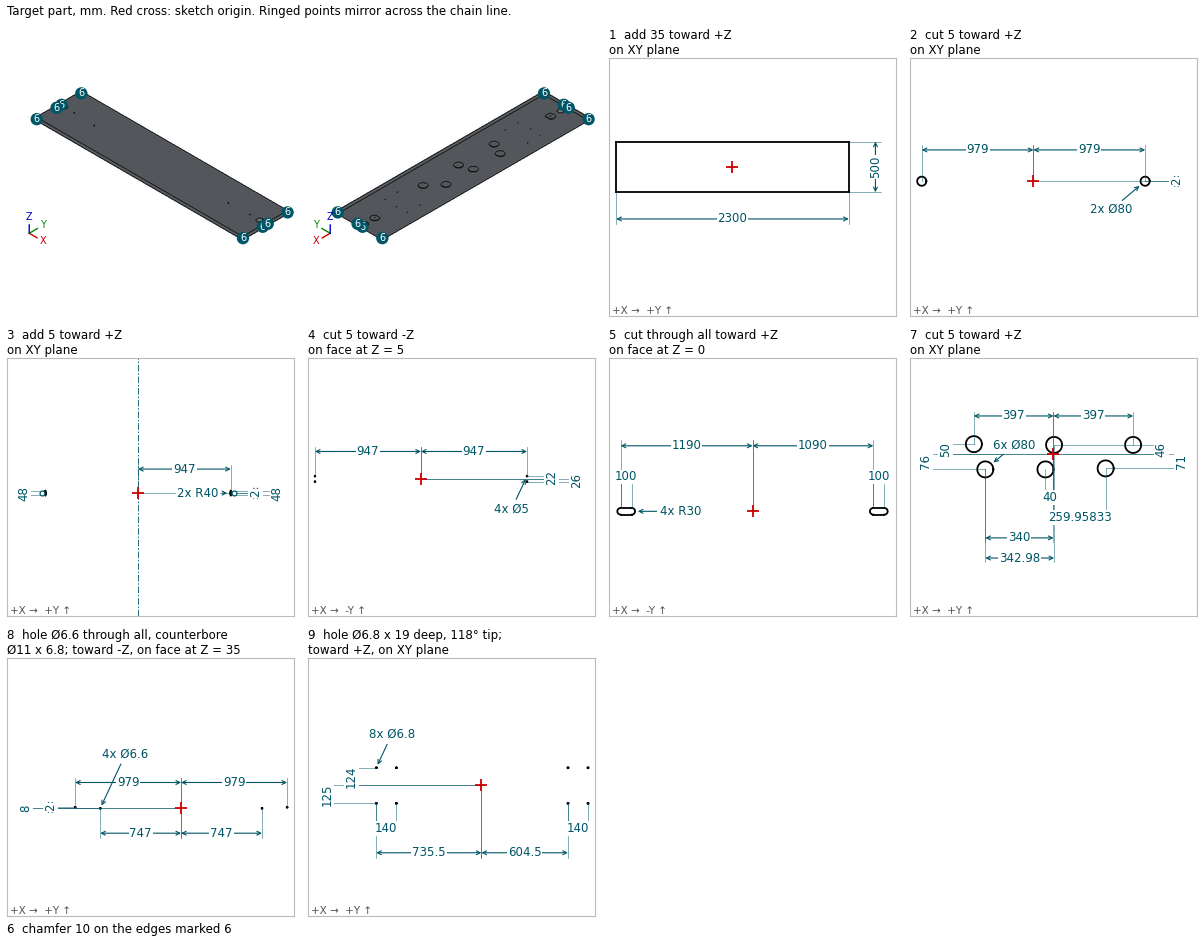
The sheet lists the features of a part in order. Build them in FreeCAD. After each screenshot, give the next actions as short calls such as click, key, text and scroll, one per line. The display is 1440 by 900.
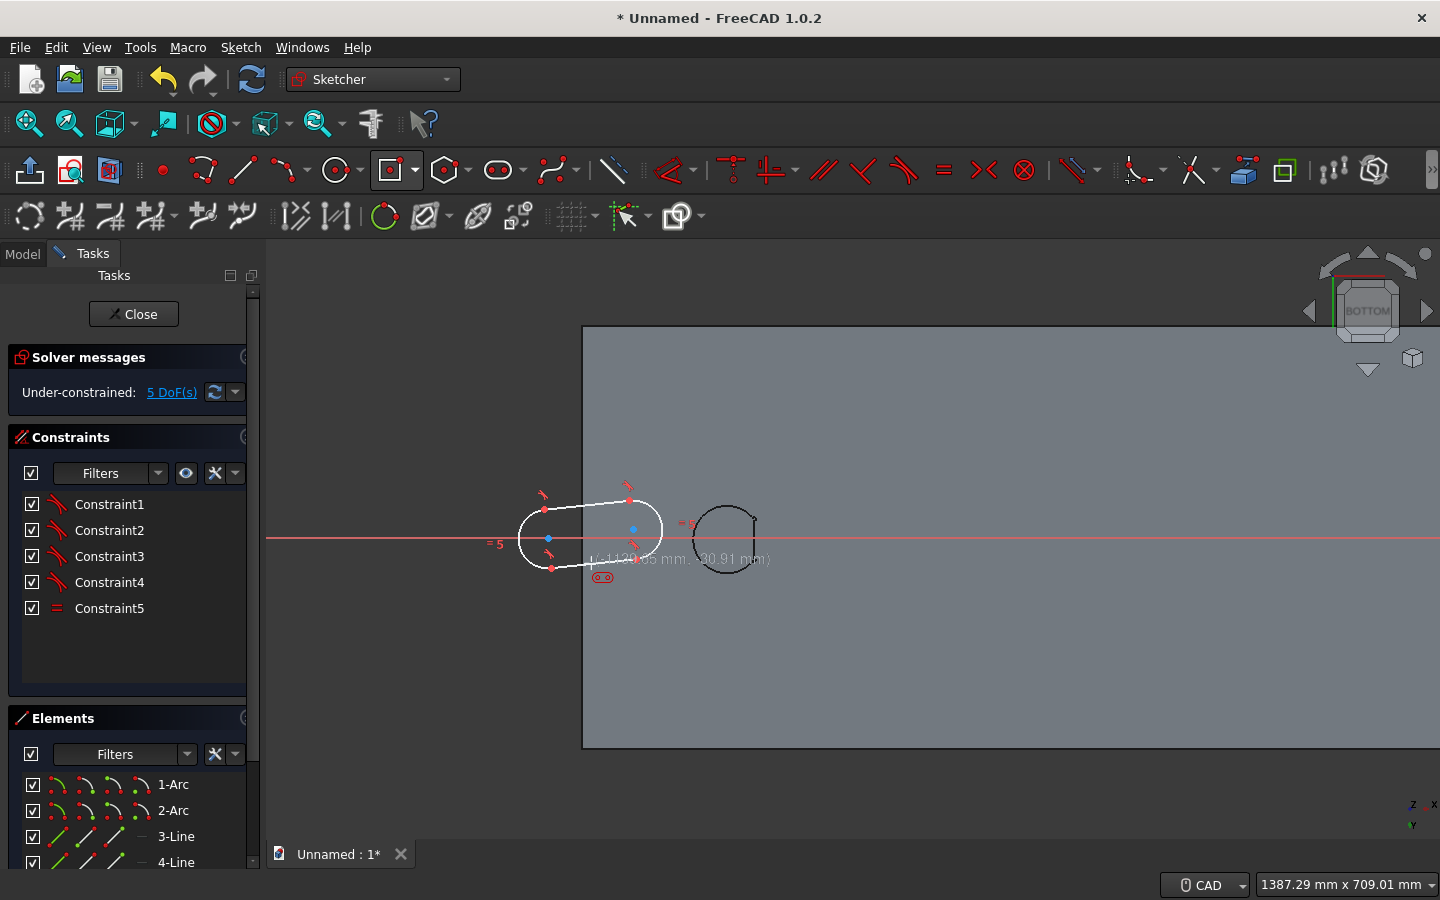
scroll(336, 540, down, 5)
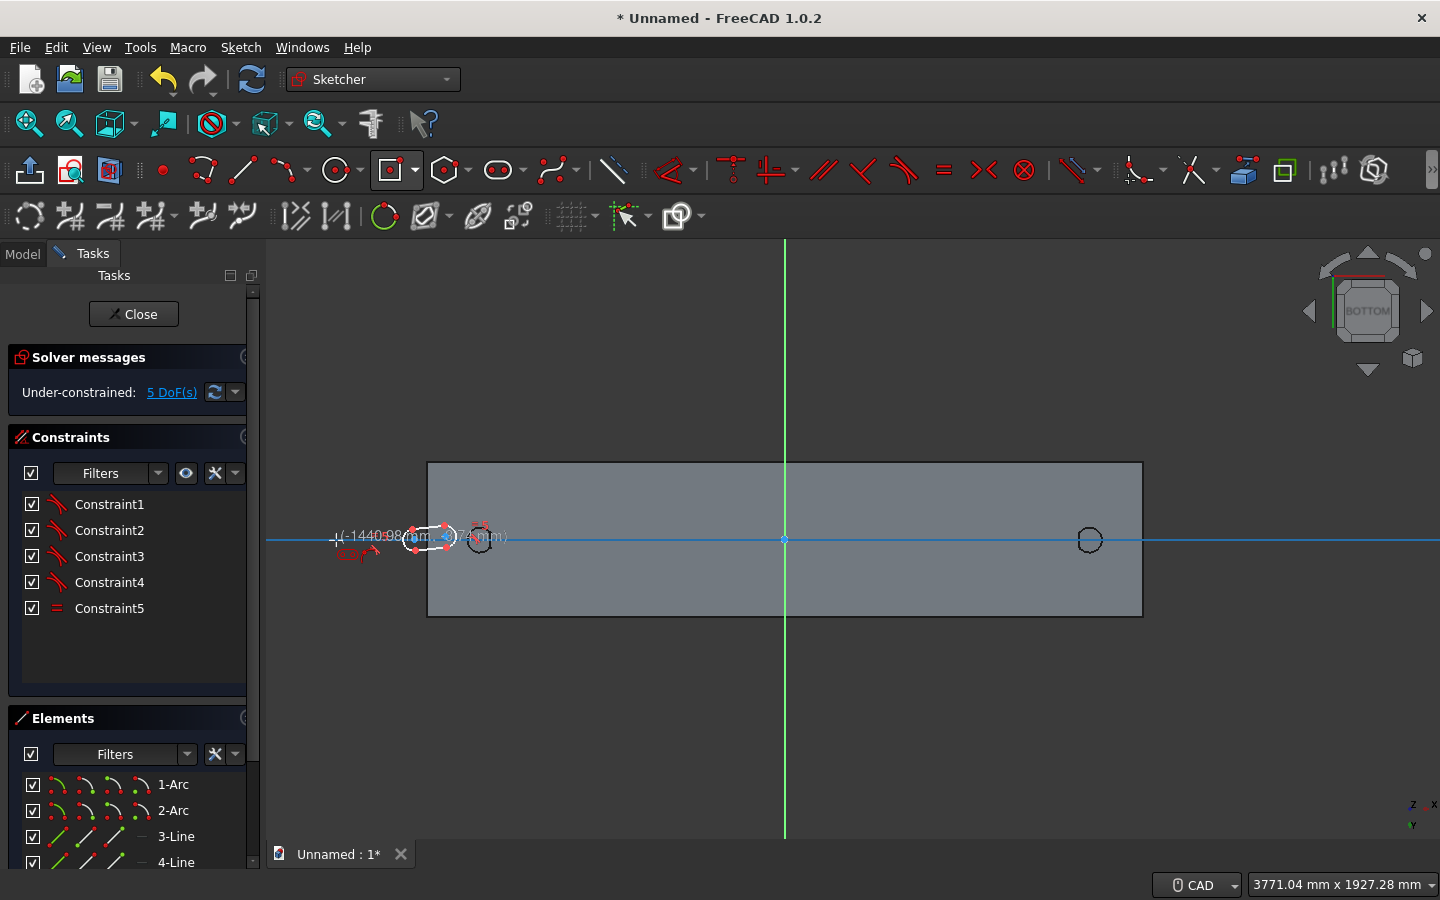
scroll(1124, 540, up, 5)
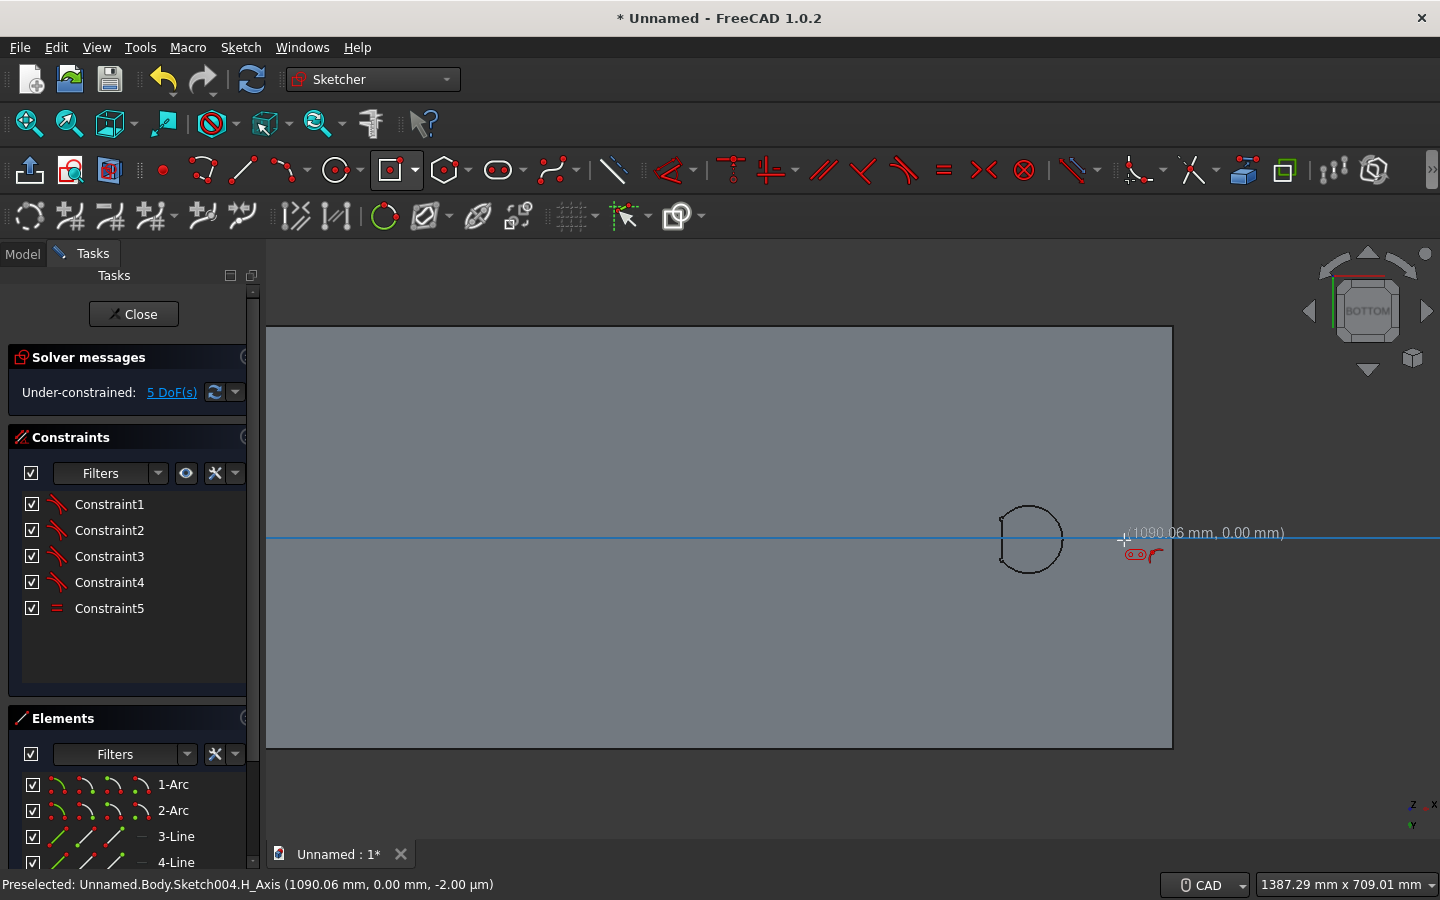
click(1123, 538)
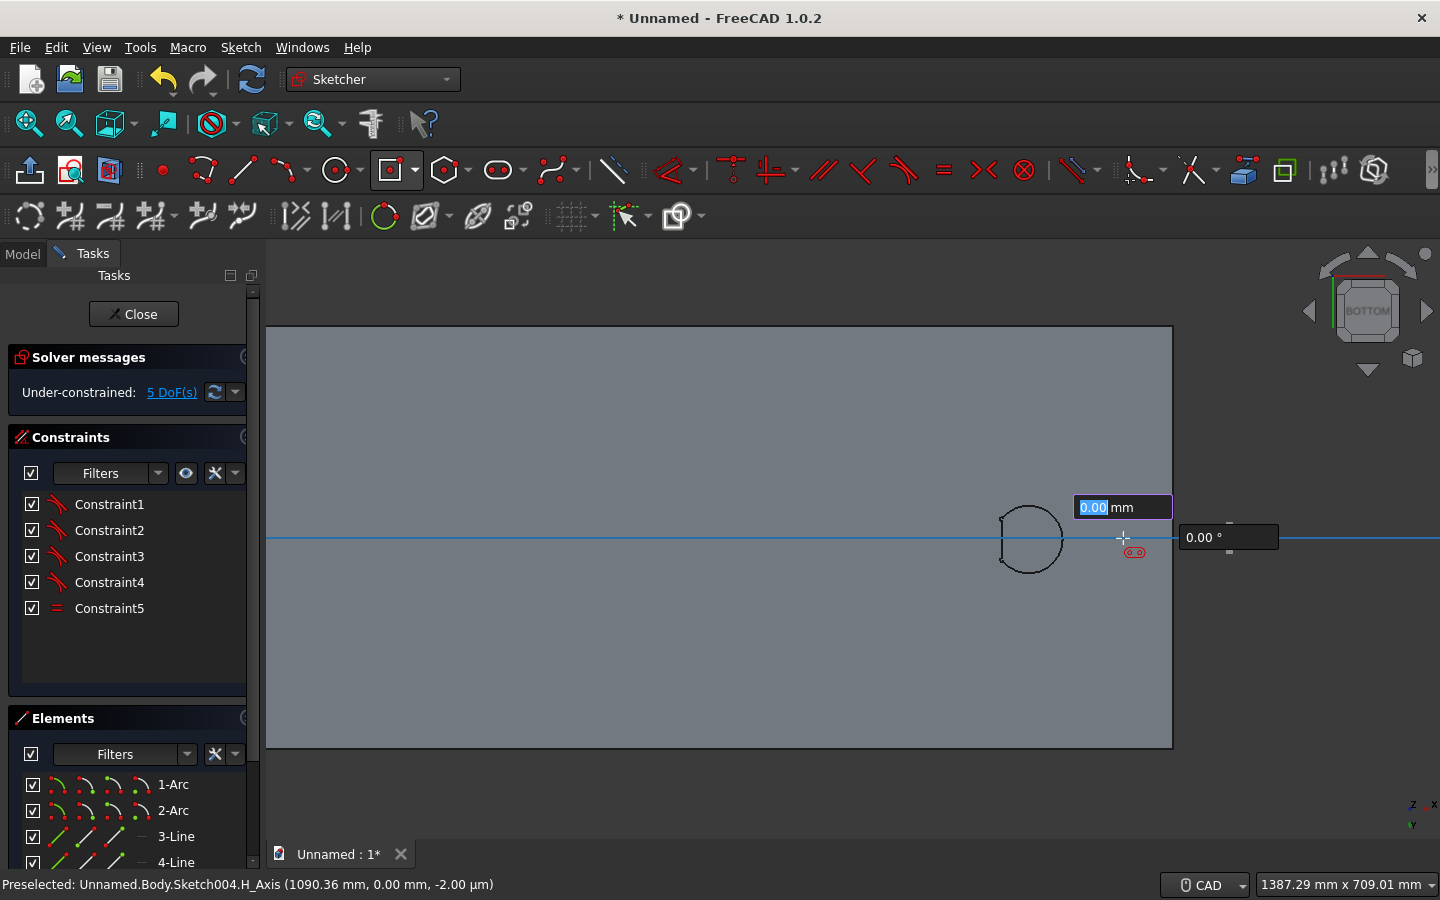
click(1207, 529)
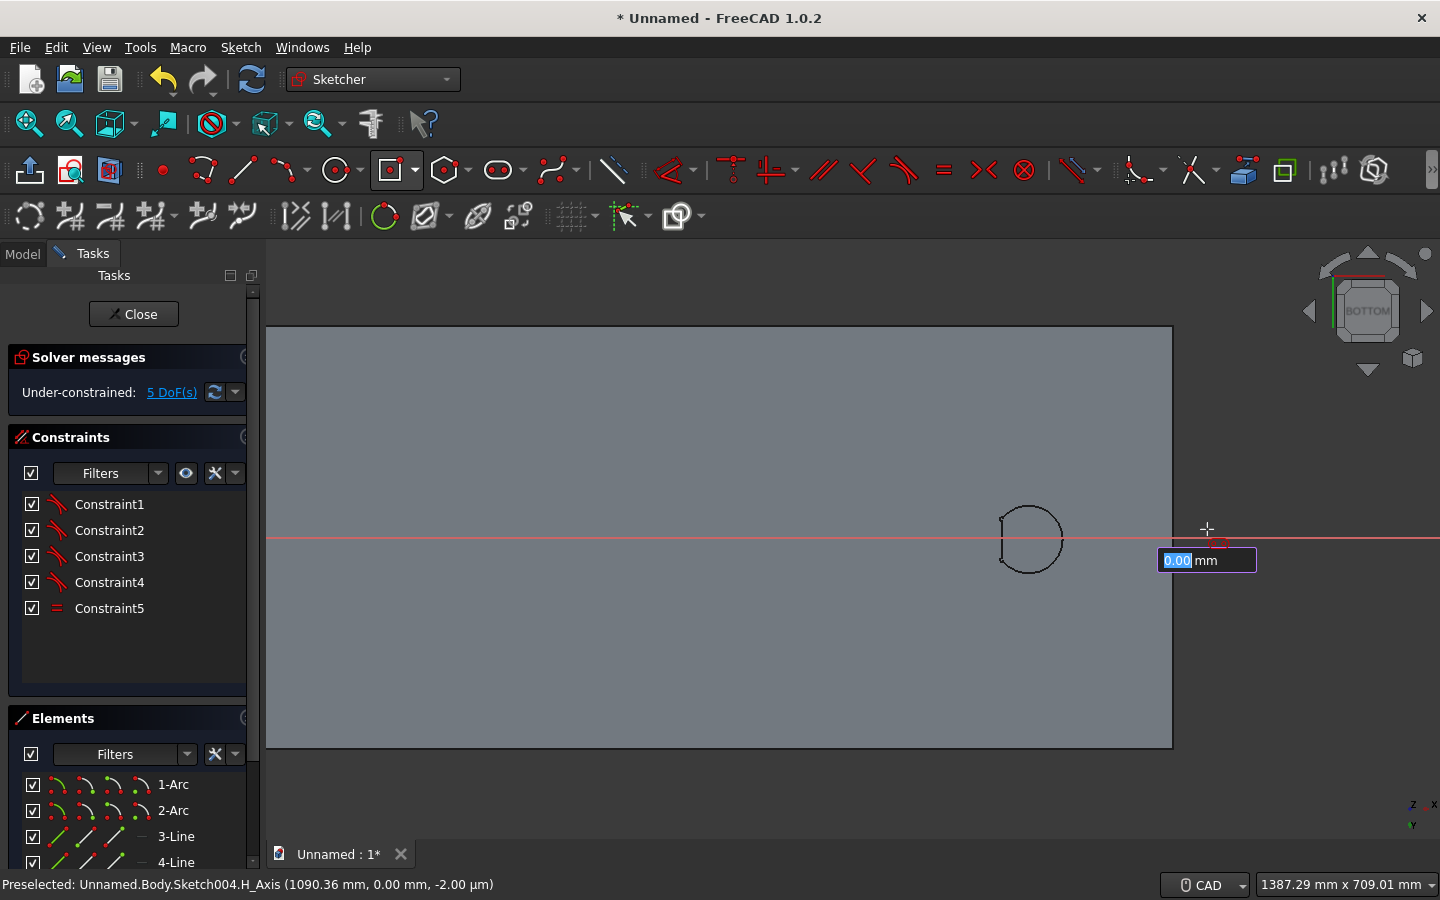
click(1165, 563)
key(Escape)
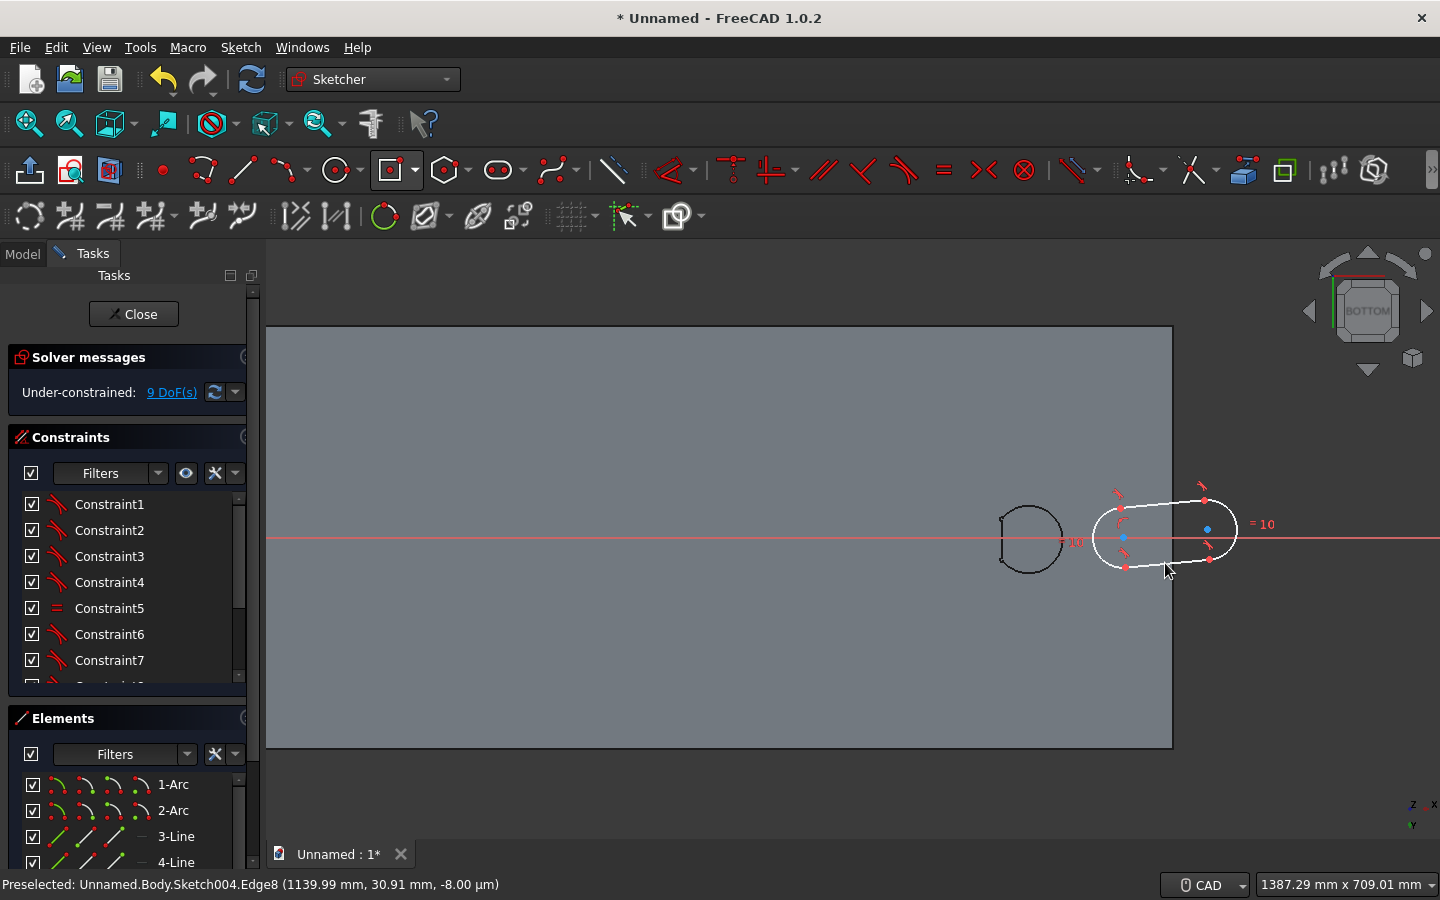
scroll(1125, 540, down, 5)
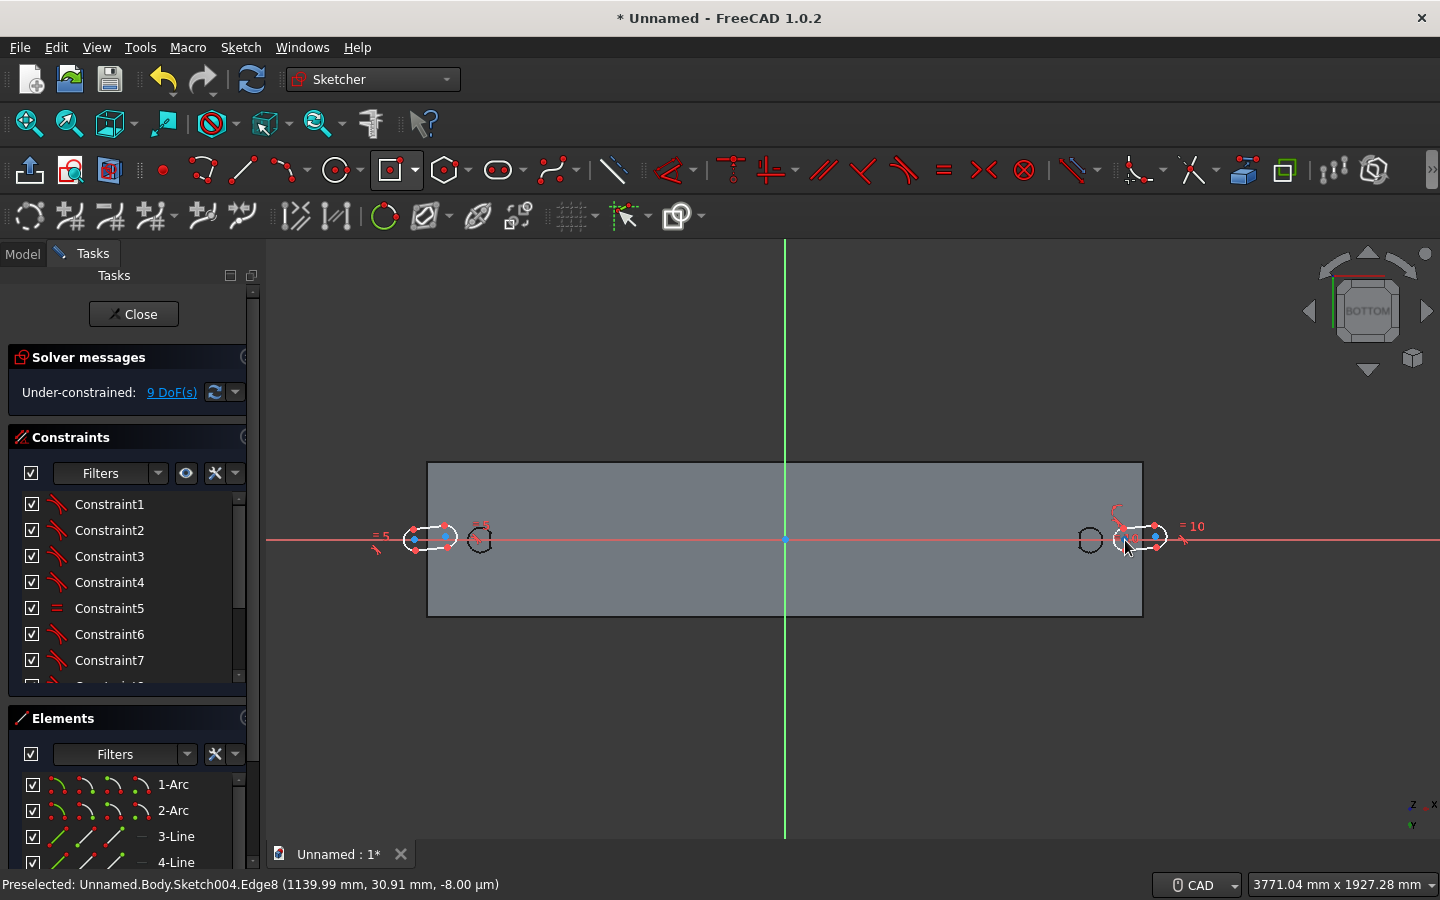
scroll(423, 528, up, 2)